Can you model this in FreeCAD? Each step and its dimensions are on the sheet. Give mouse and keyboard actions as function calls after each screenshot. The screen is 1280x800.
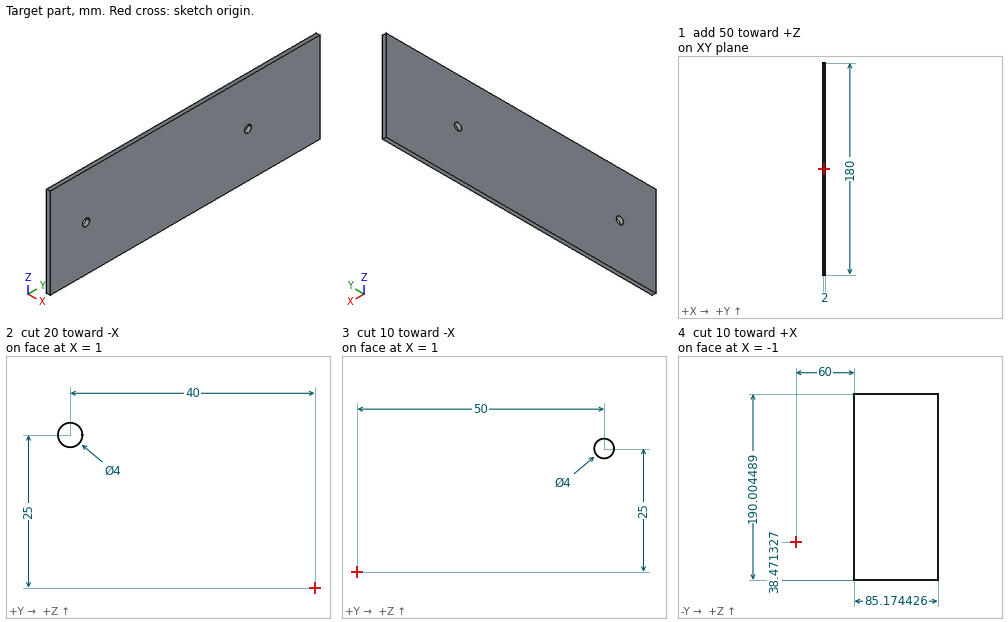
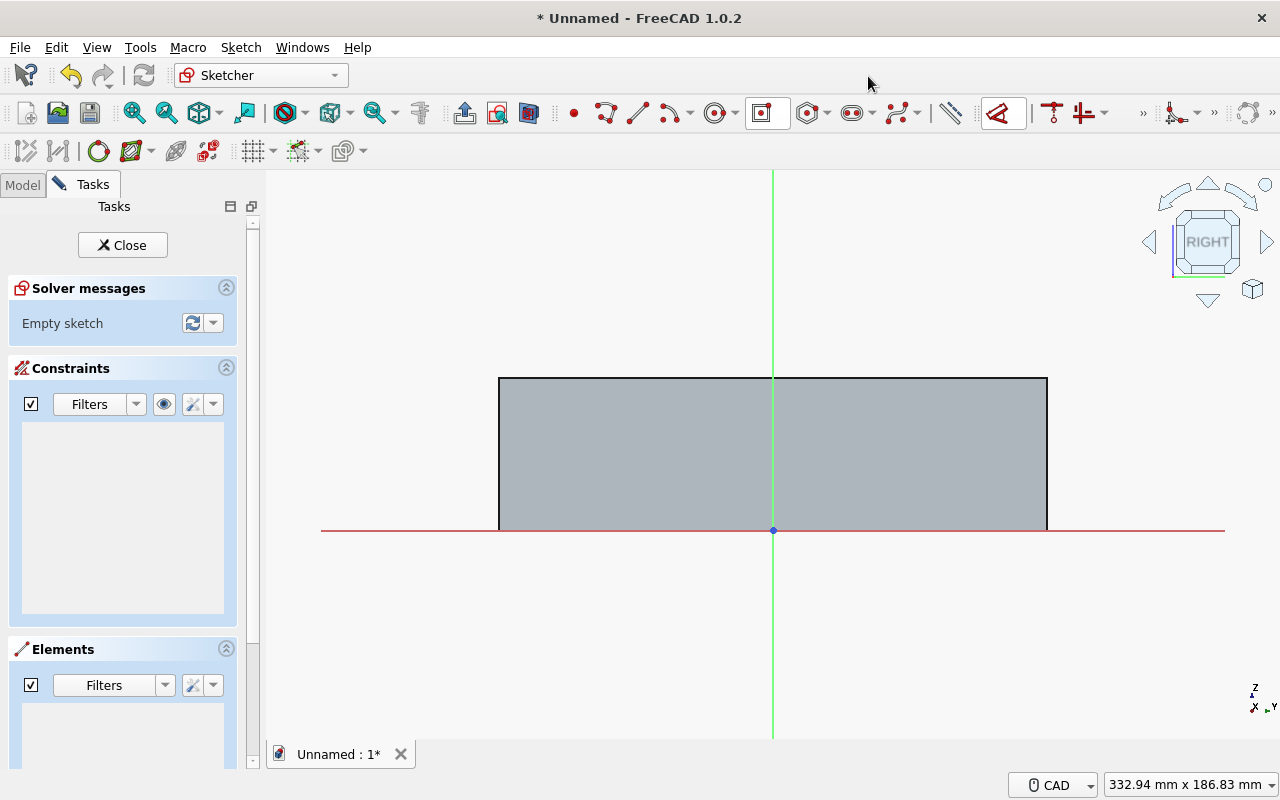
scroll(648, 455, up, 15)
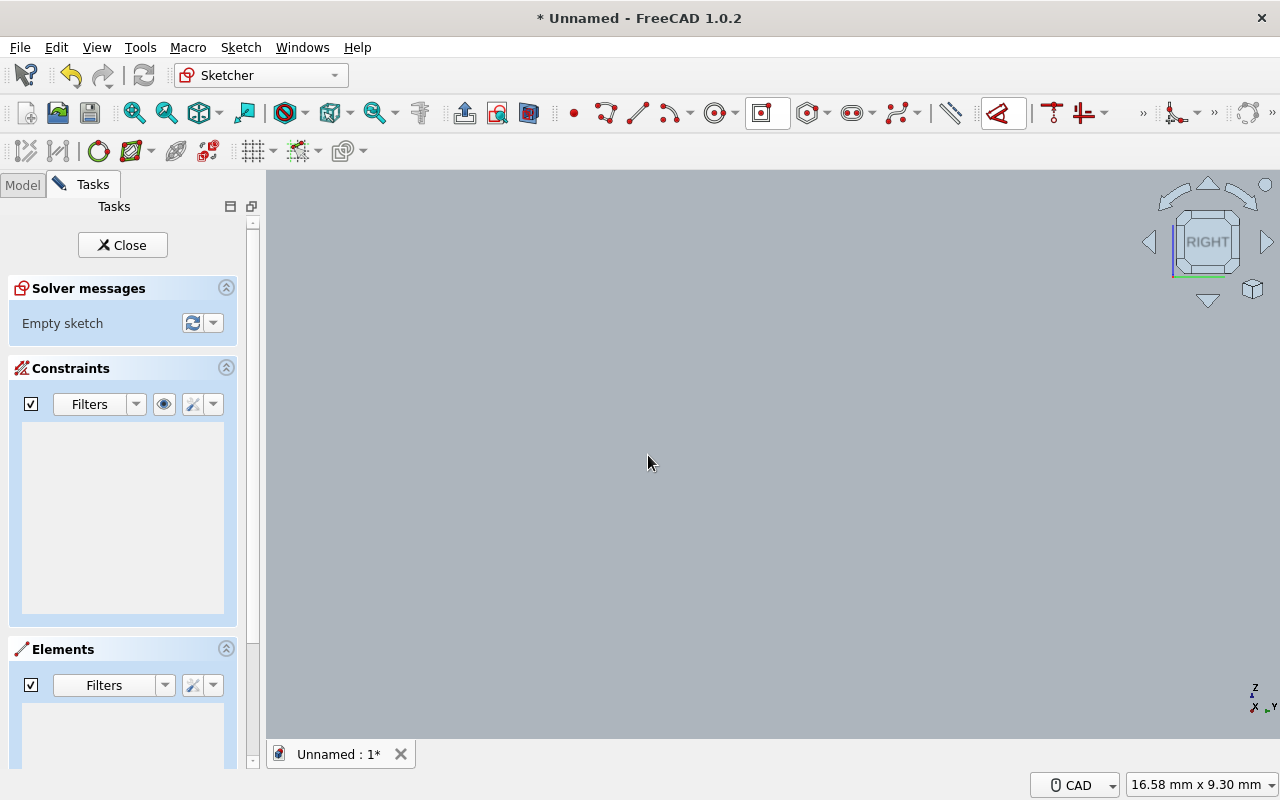
scroll(705, 397, up, 2)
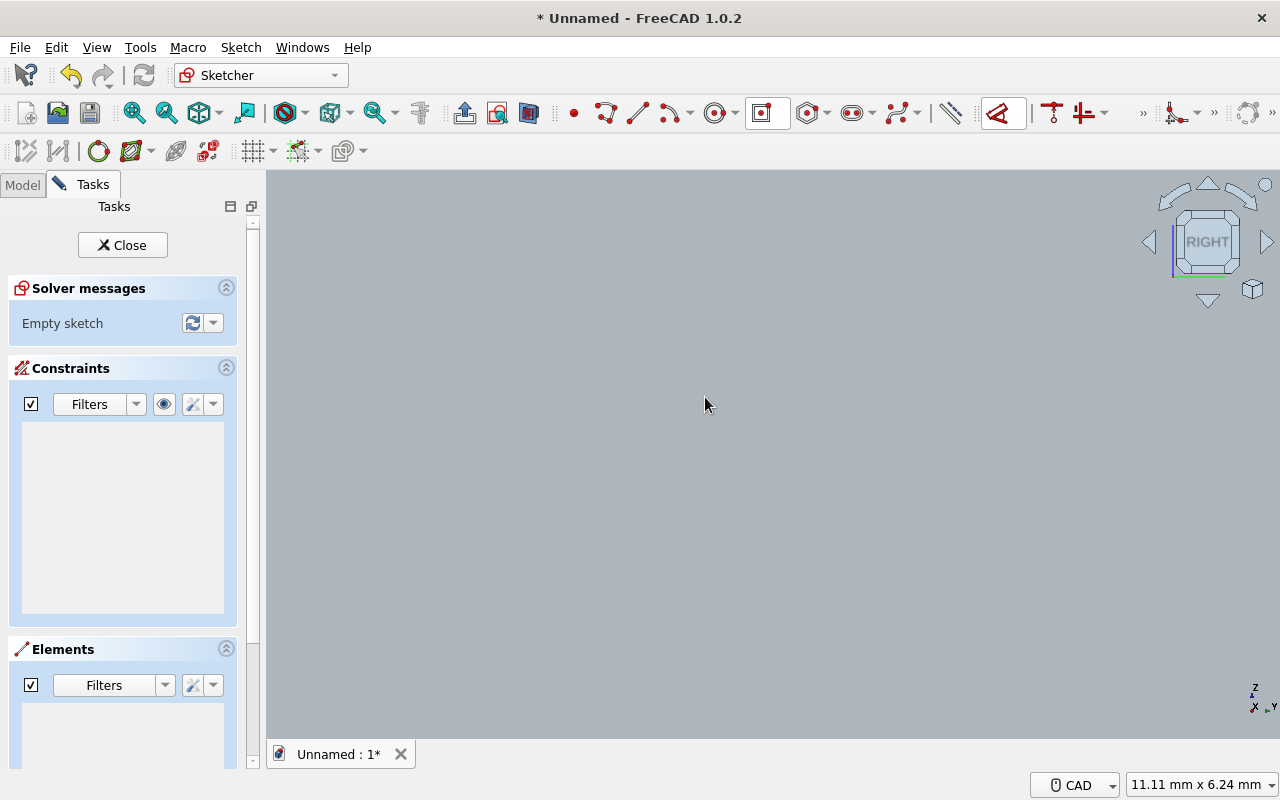
click(716, 114)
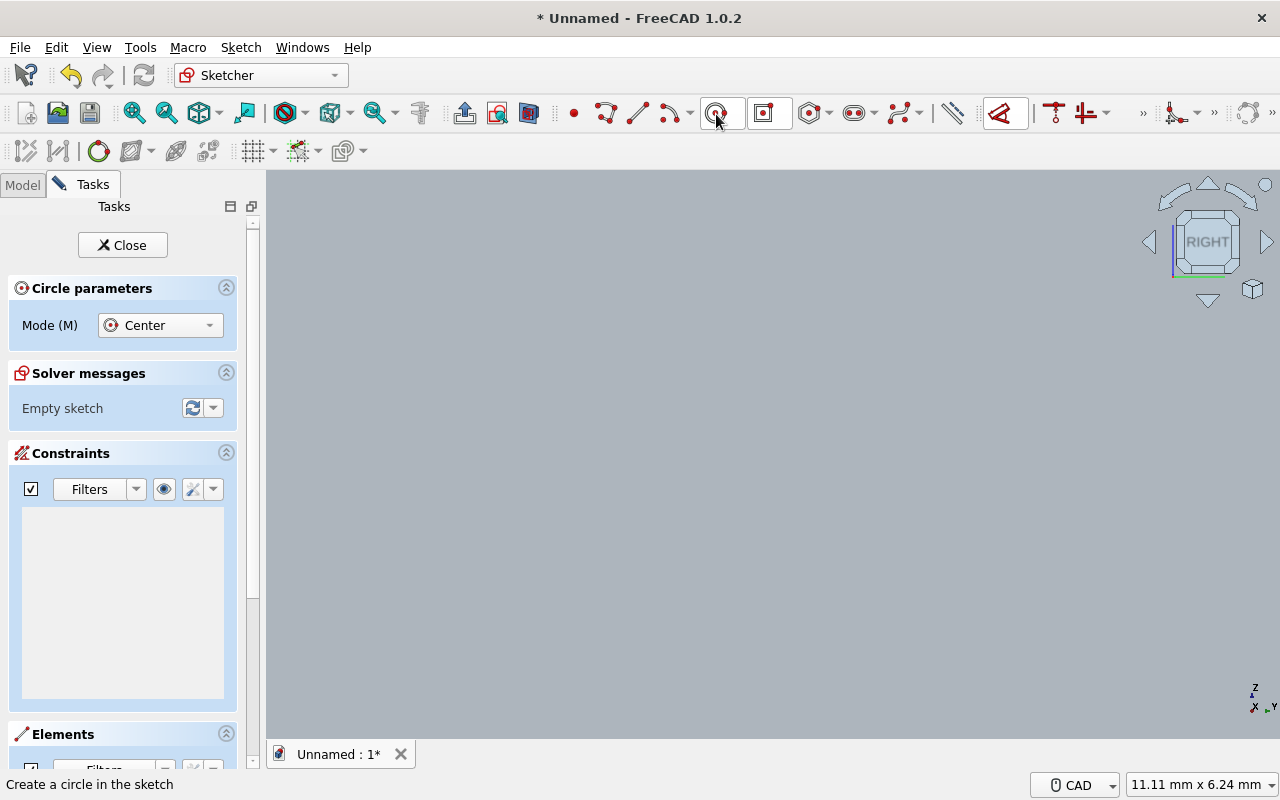
click(704, 454)
click(833, 325)
key(Escape)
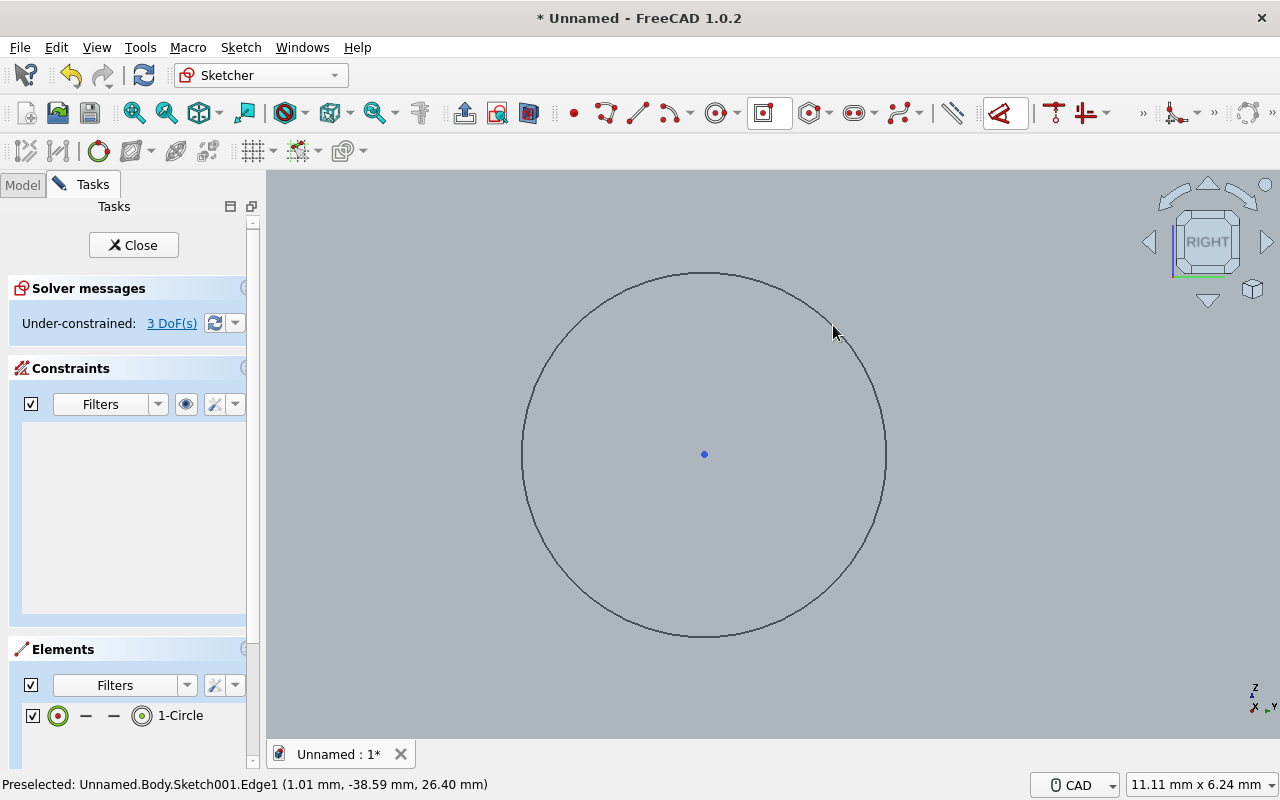
click(833, 326)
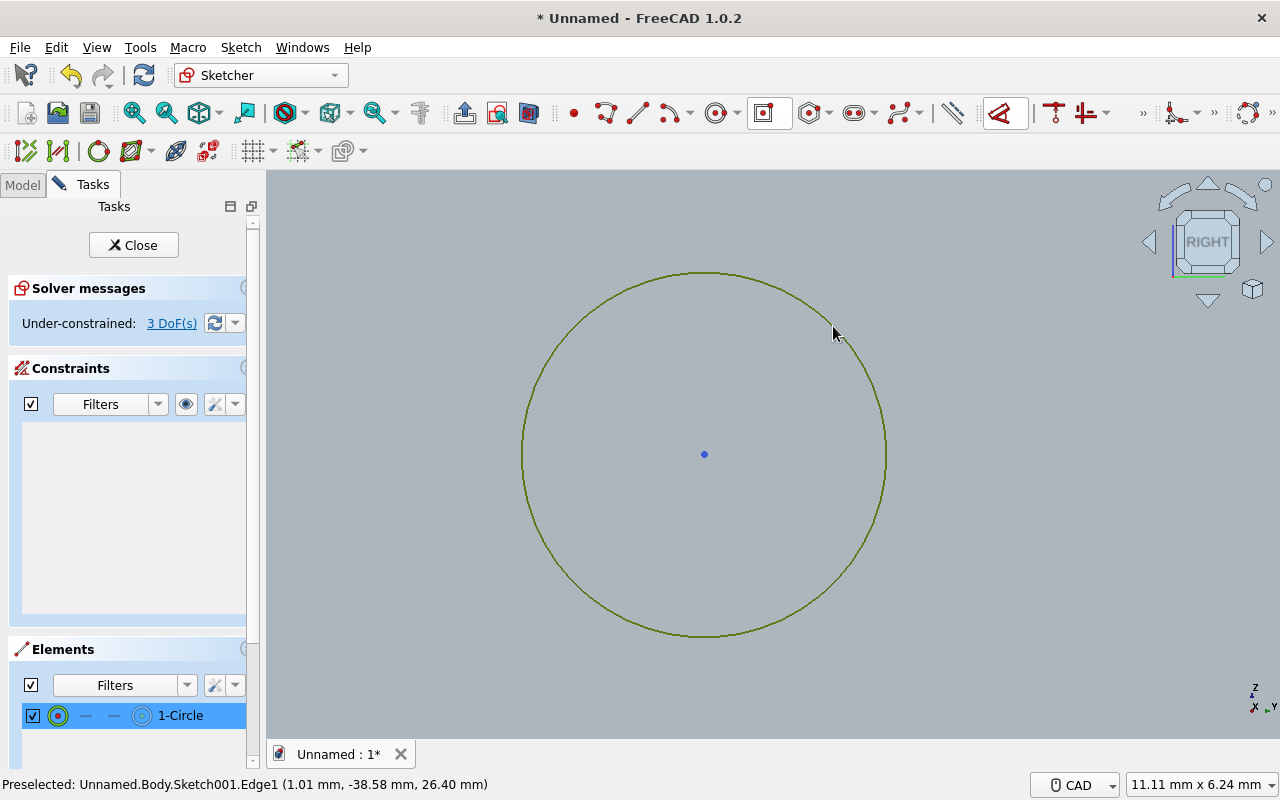
key(k)
key(o)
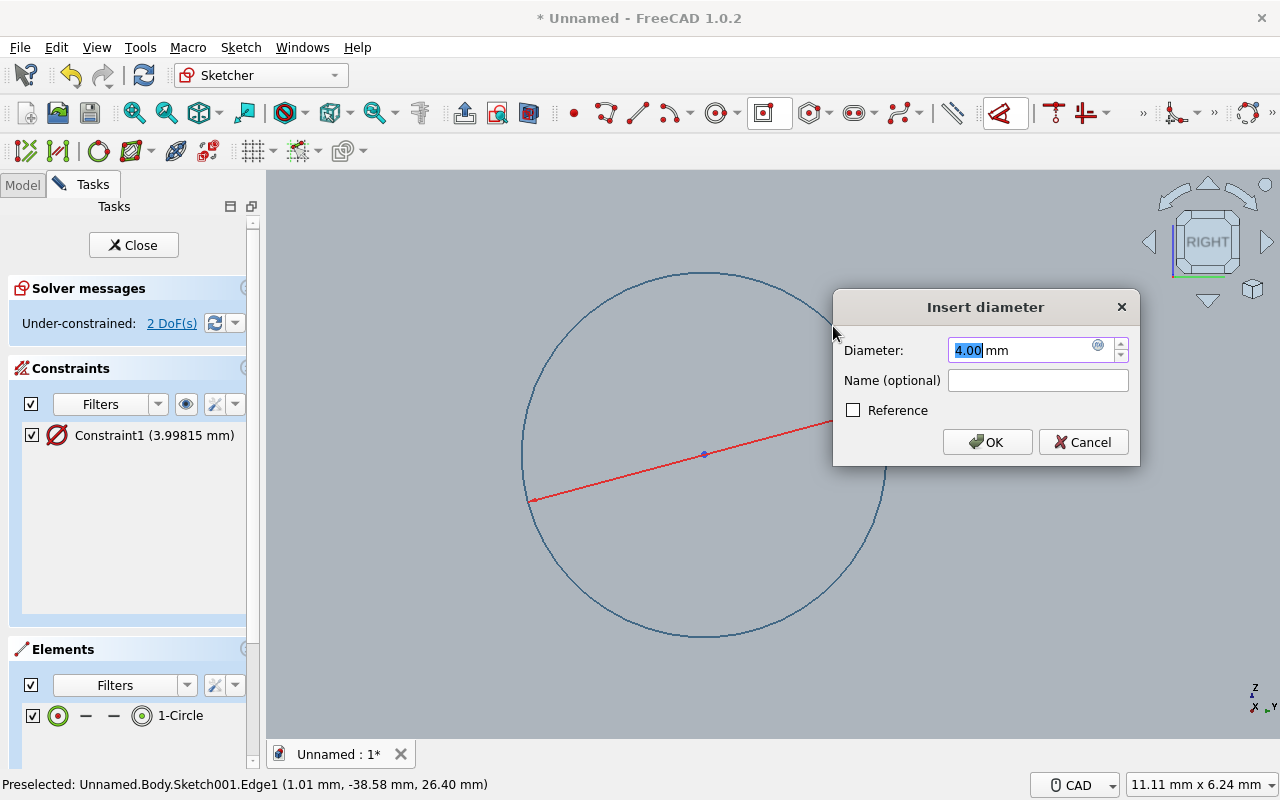
text(4)
key(Return)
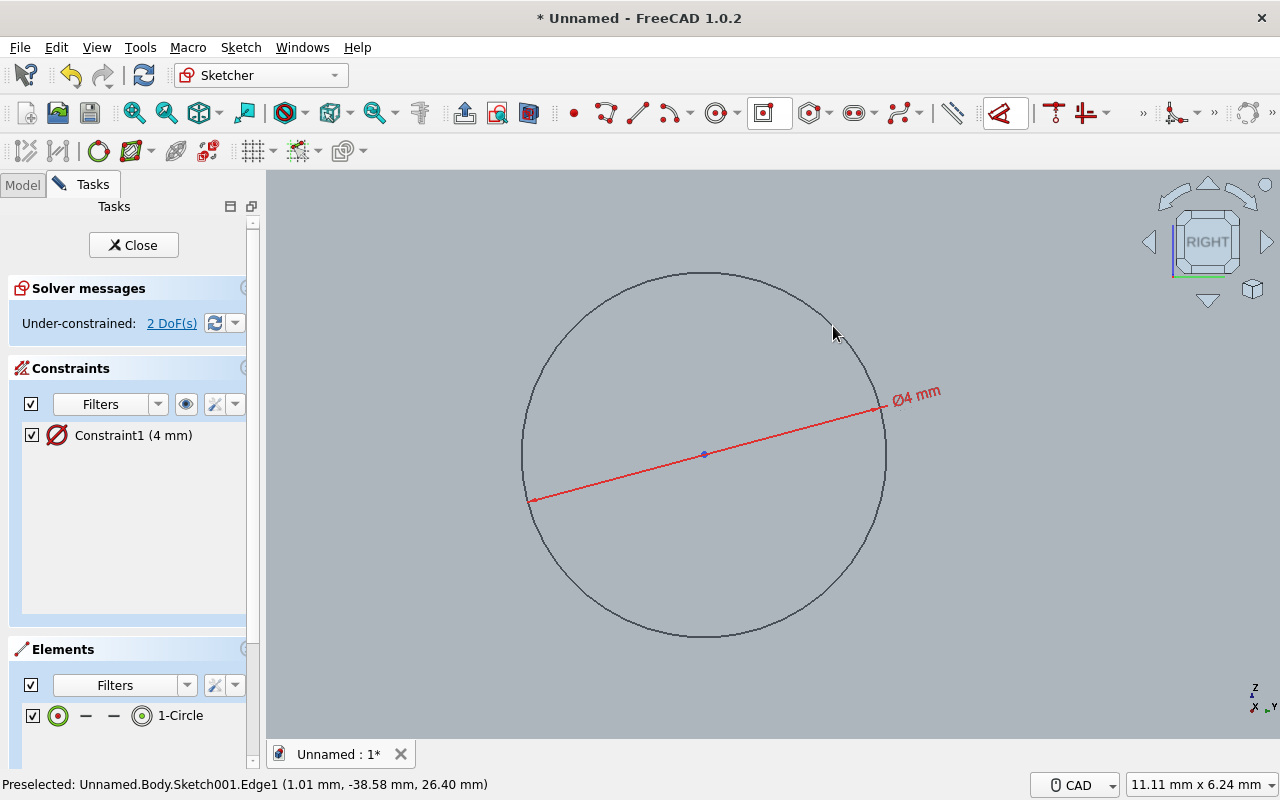
click(704, 455)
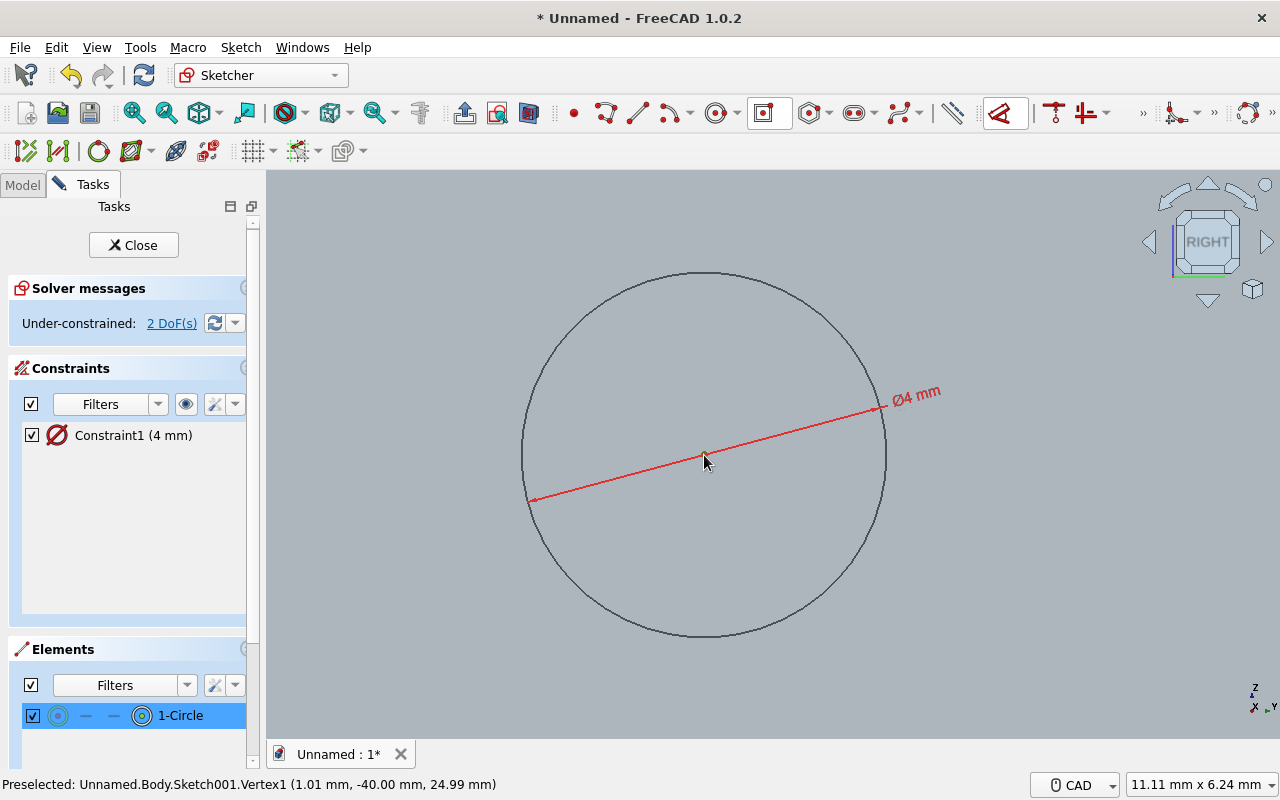
key(l)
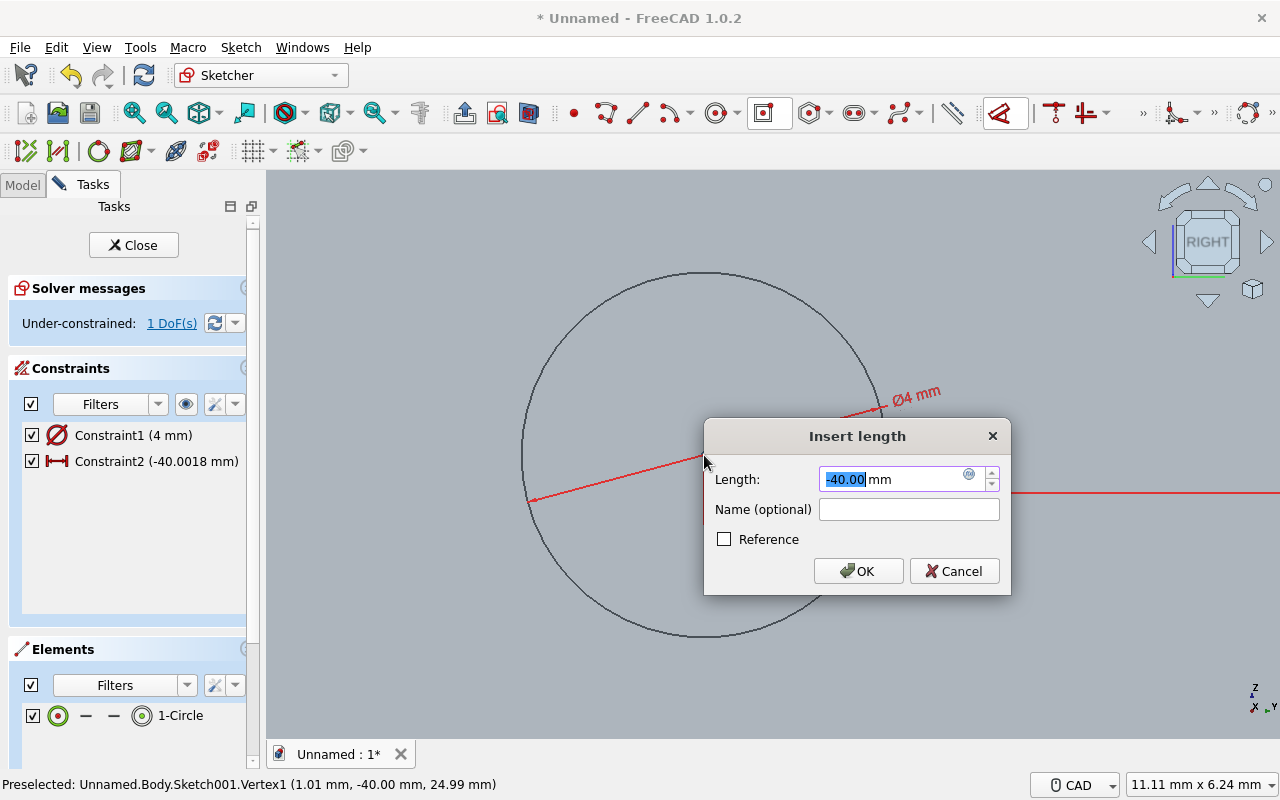
text(-40)
key(Return)